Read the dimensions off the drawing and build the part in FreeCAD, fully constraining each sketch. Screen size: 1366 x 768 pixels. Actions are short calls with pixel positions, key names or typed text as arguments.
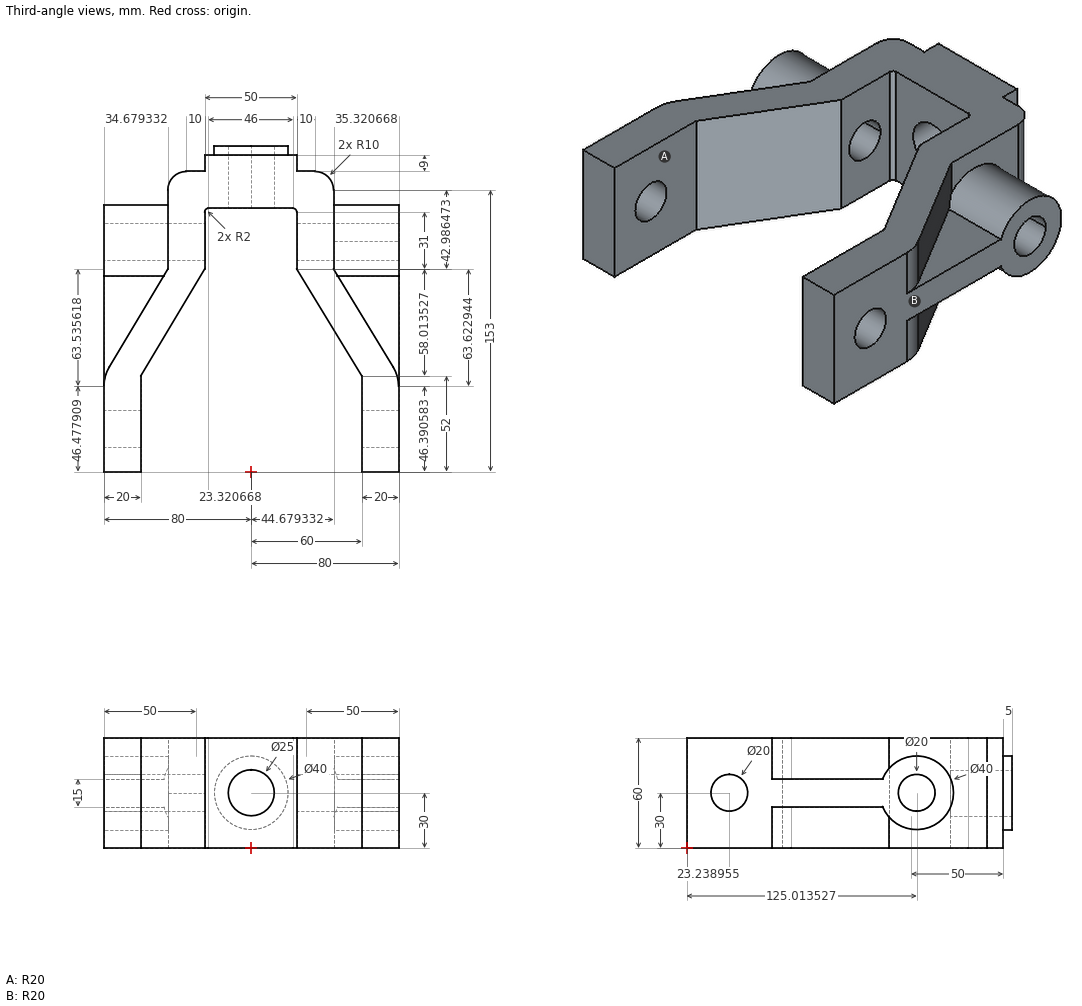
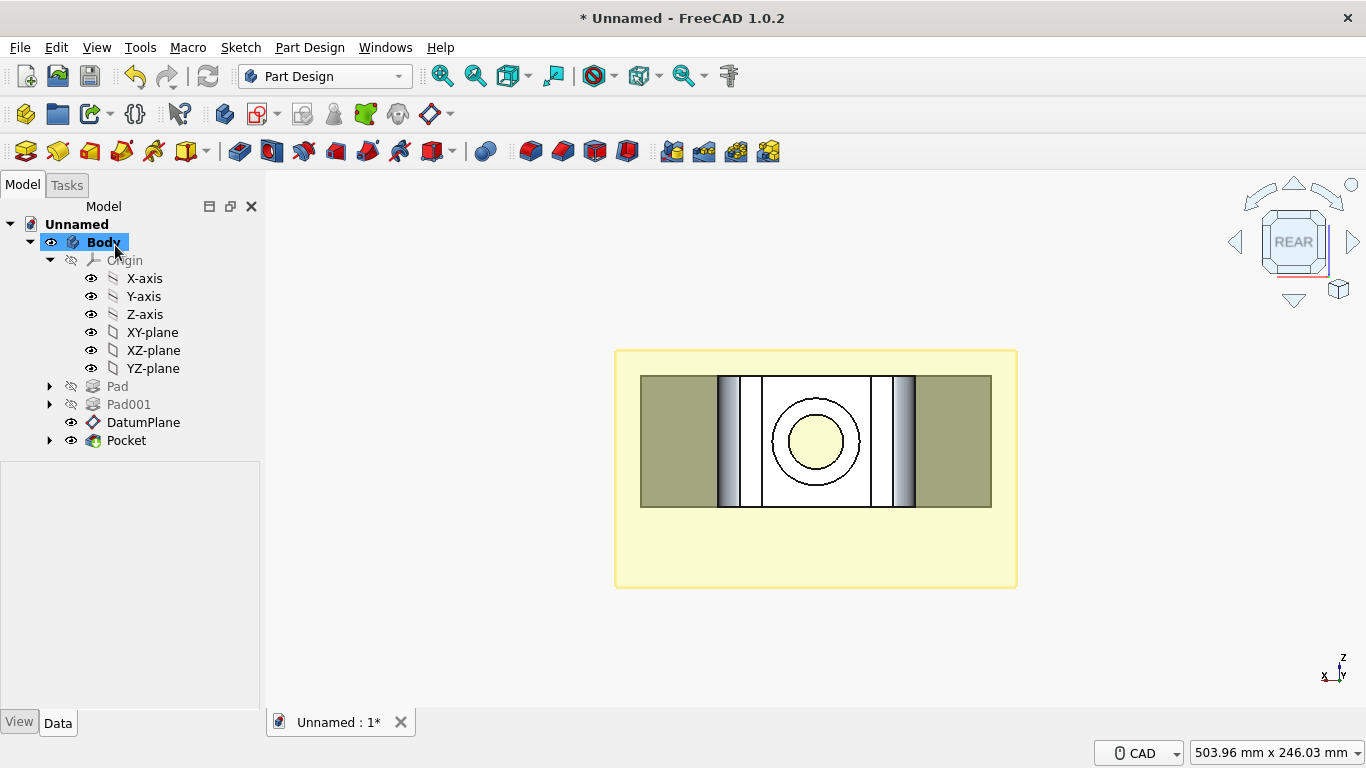
click(116, 422)
key(space)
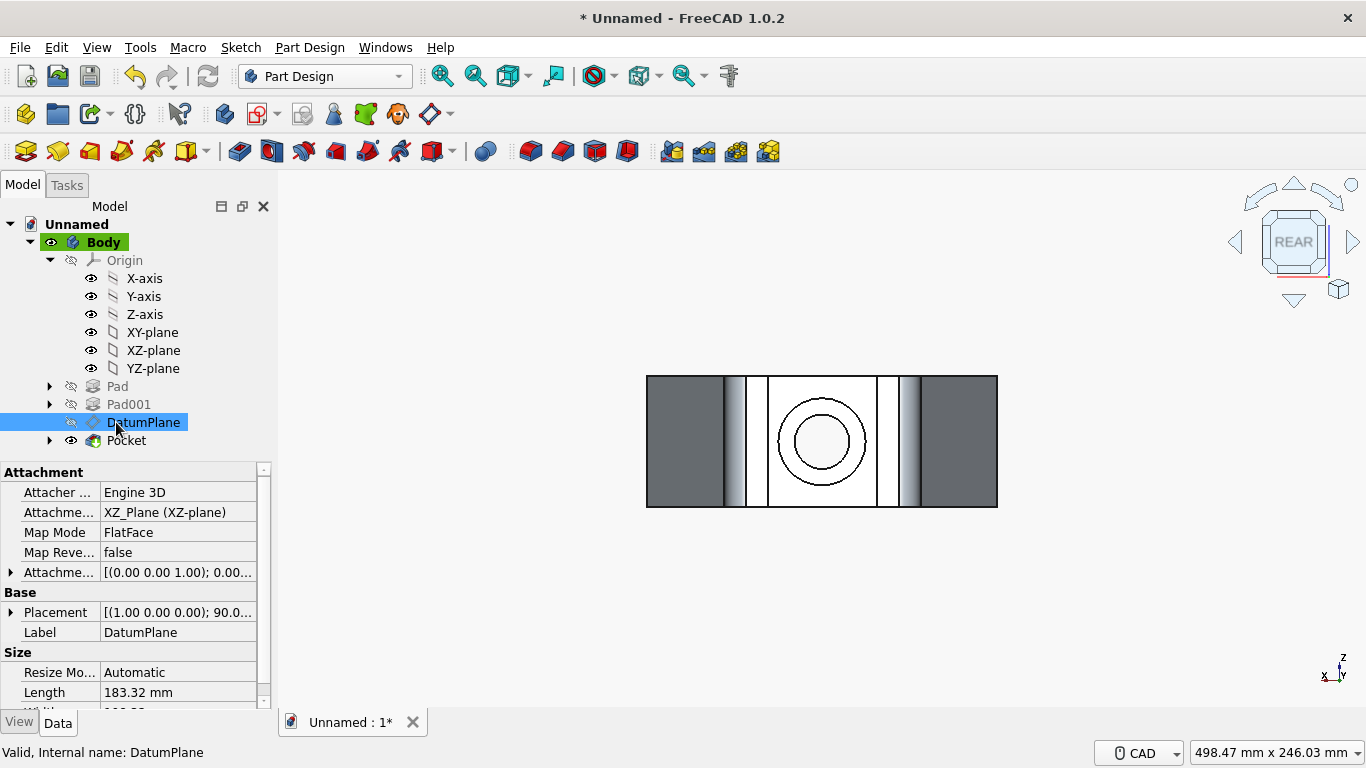
key(v)
key(f)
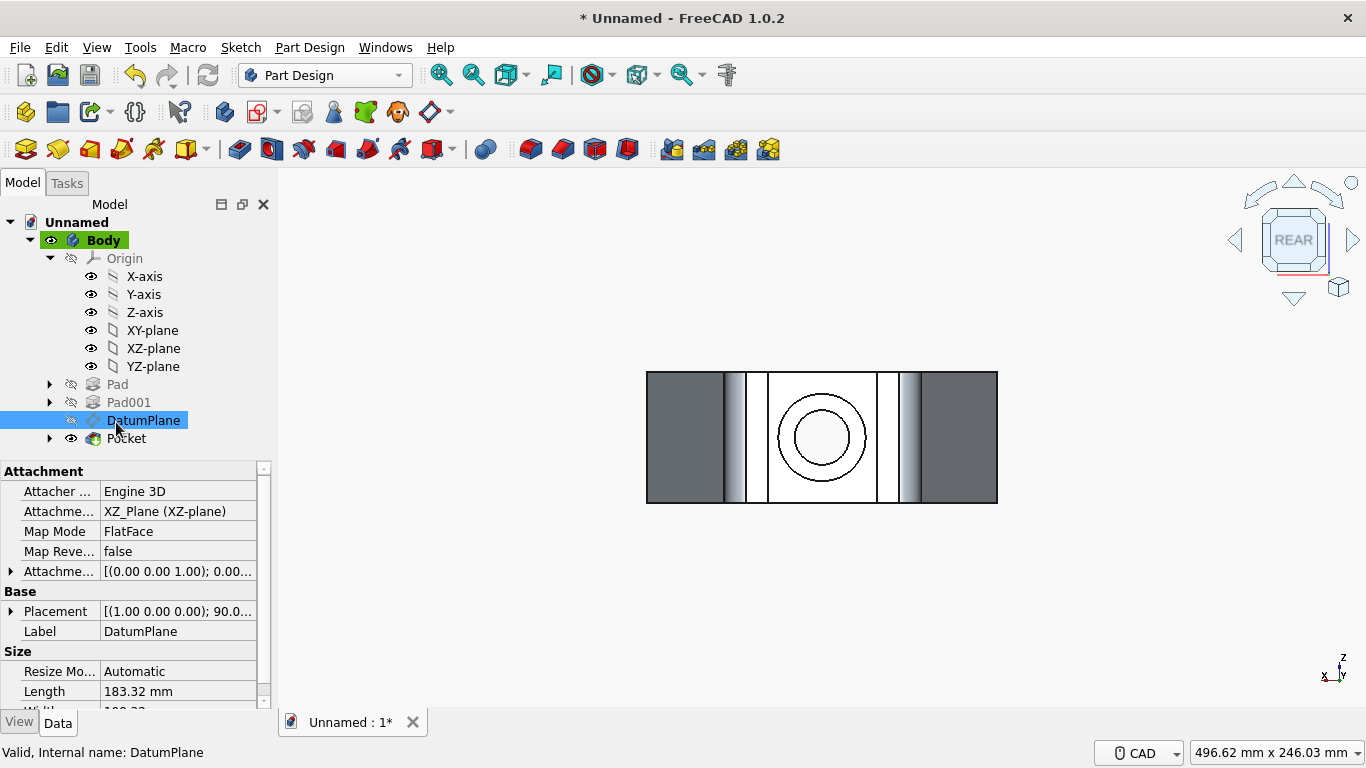
key(0)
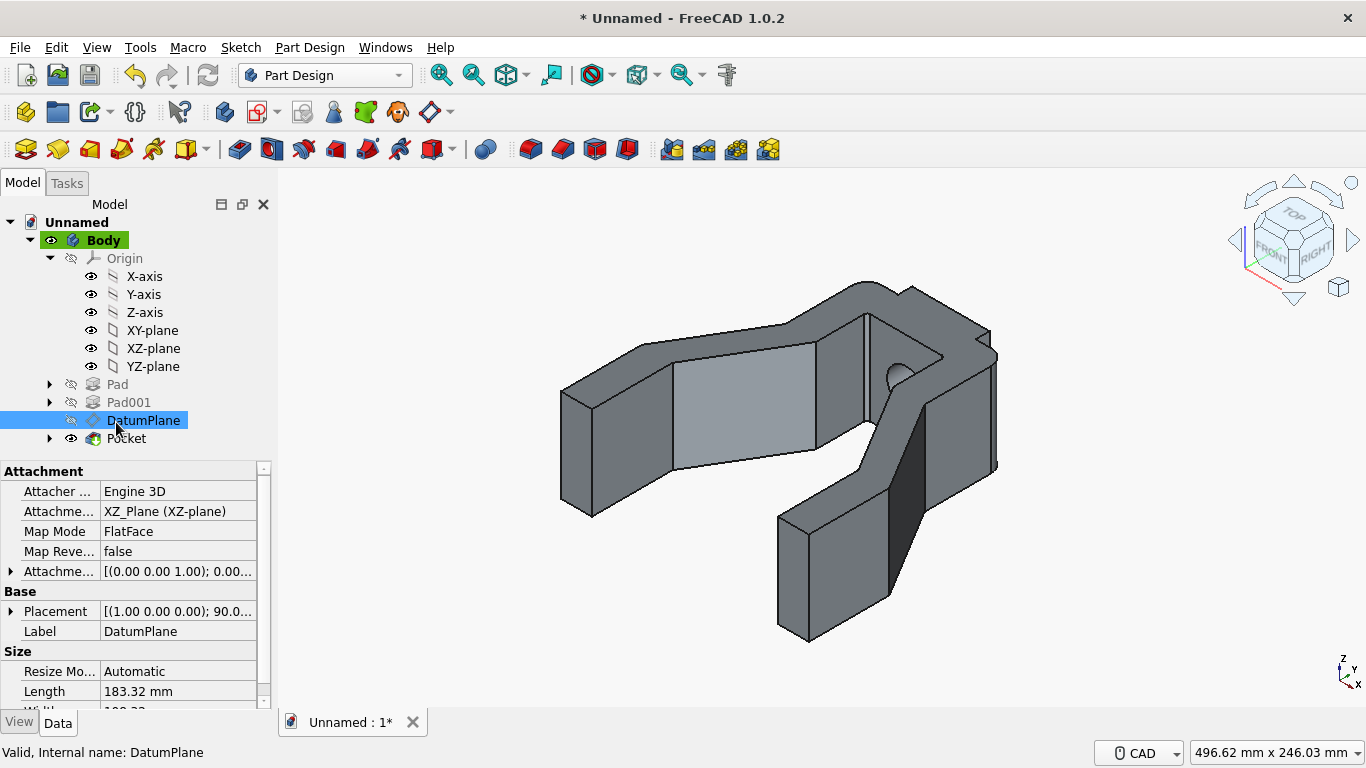
key(2)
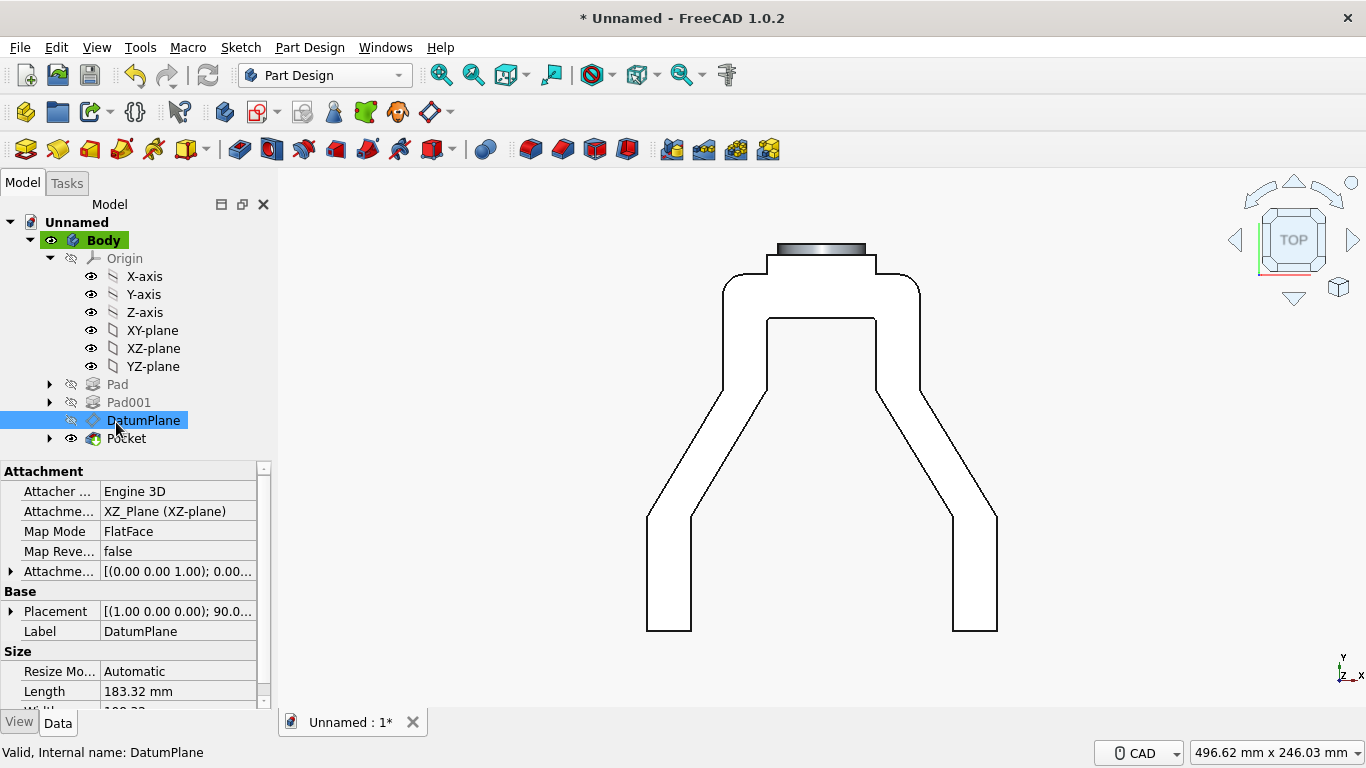
key(1)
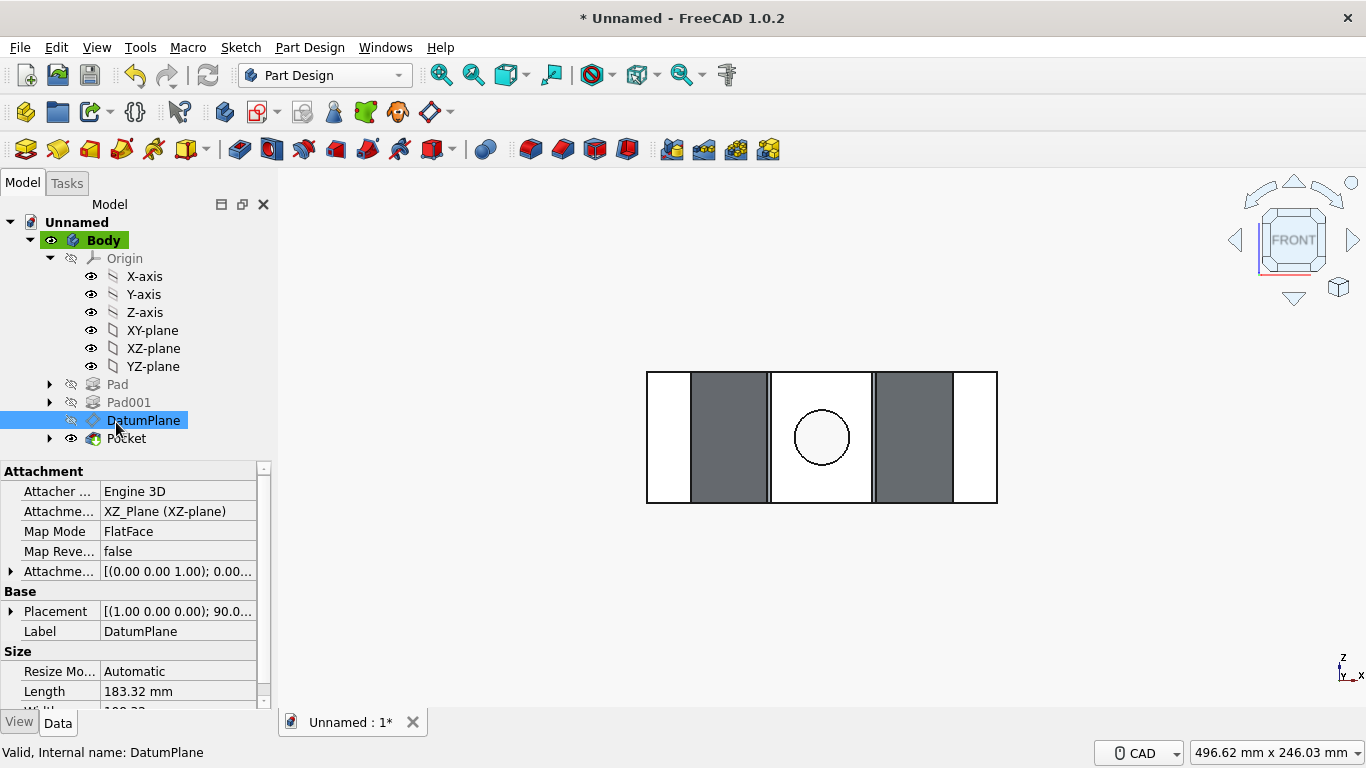
click(442, 76)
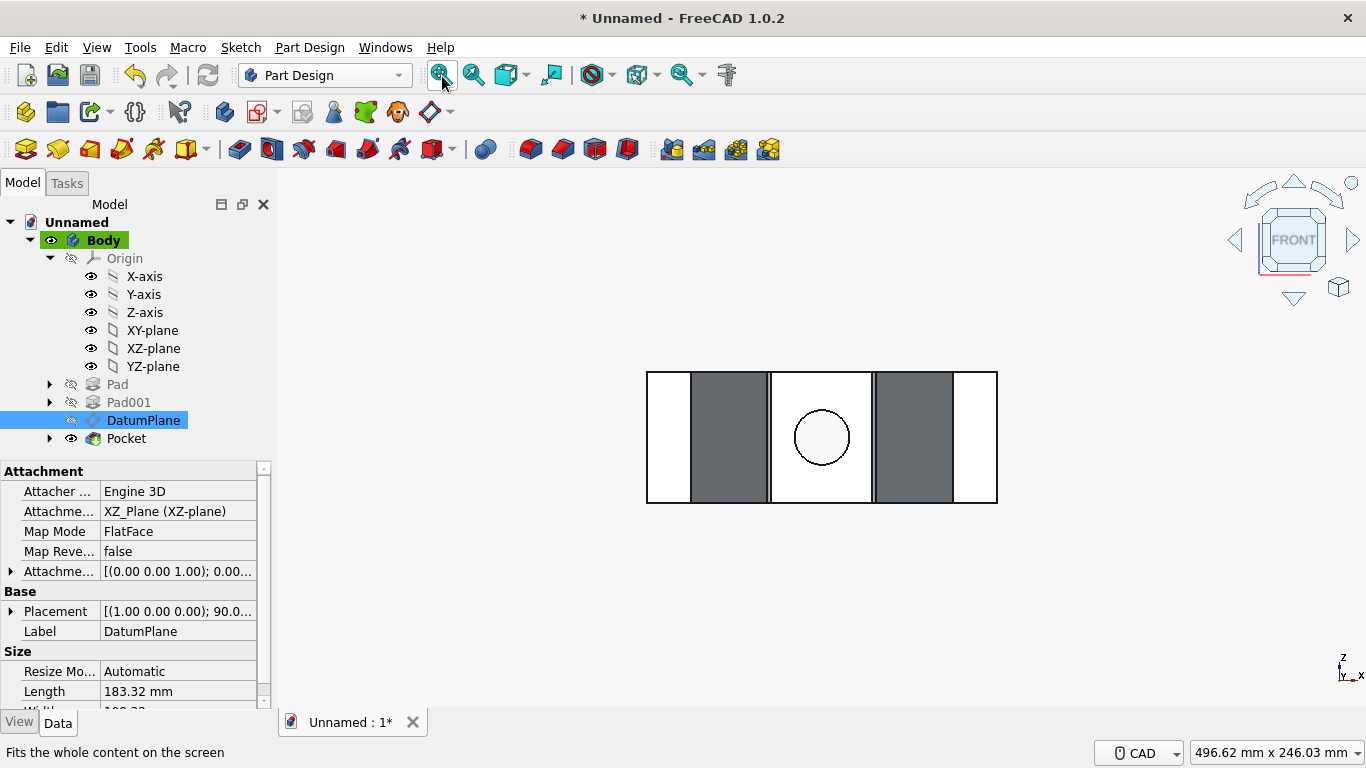
key(3)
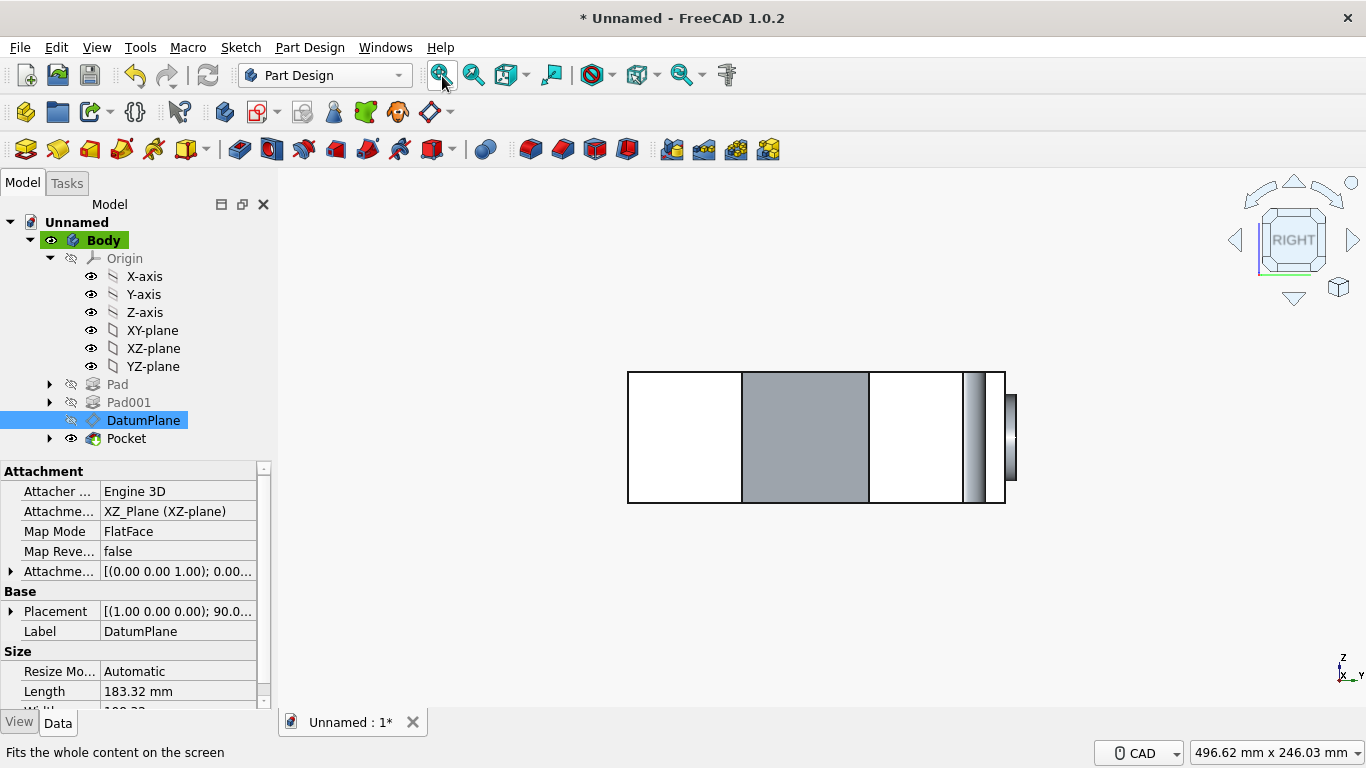
key(v)
key(f)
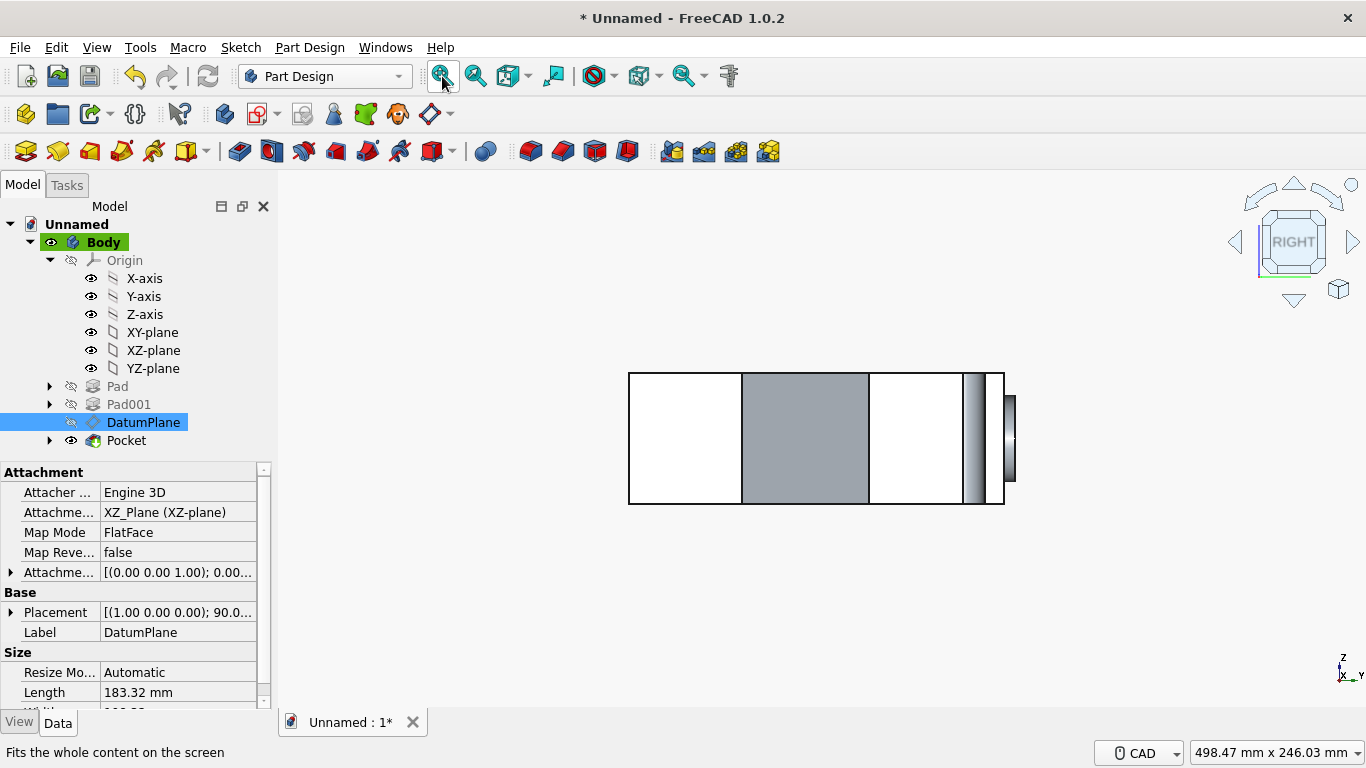
key(5)